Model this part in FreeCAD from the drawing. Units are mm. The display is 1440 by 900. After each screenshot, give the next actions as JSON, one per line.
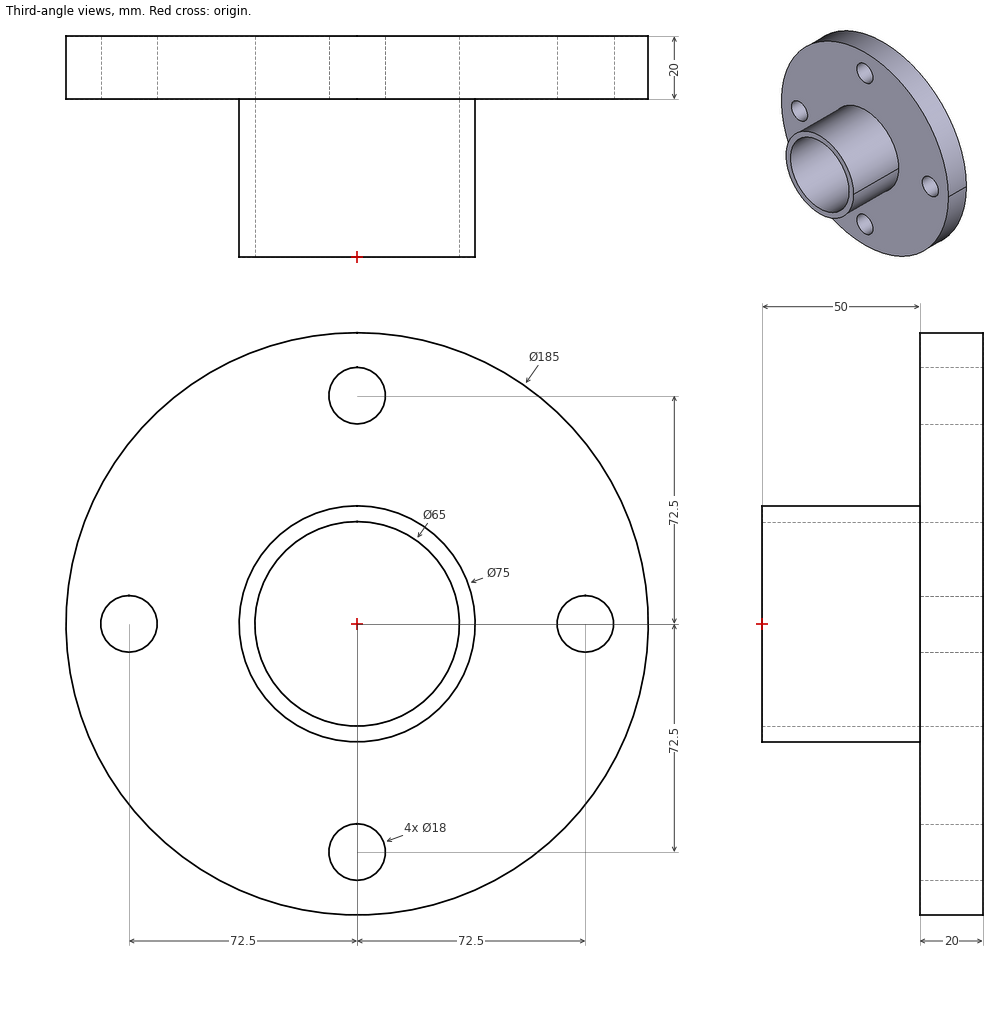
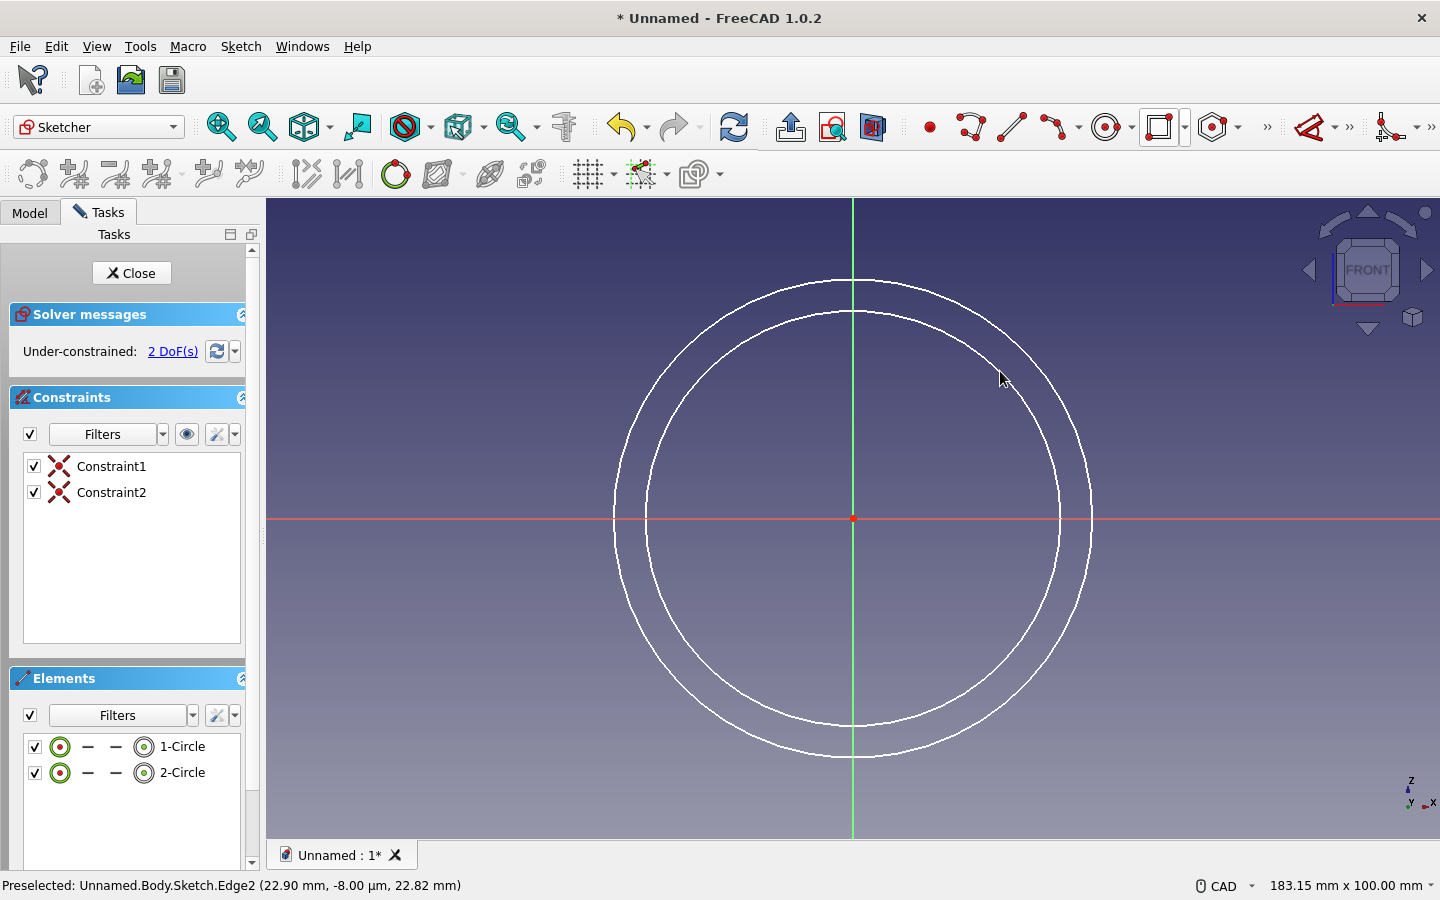
{"action": "key", "text": "d"}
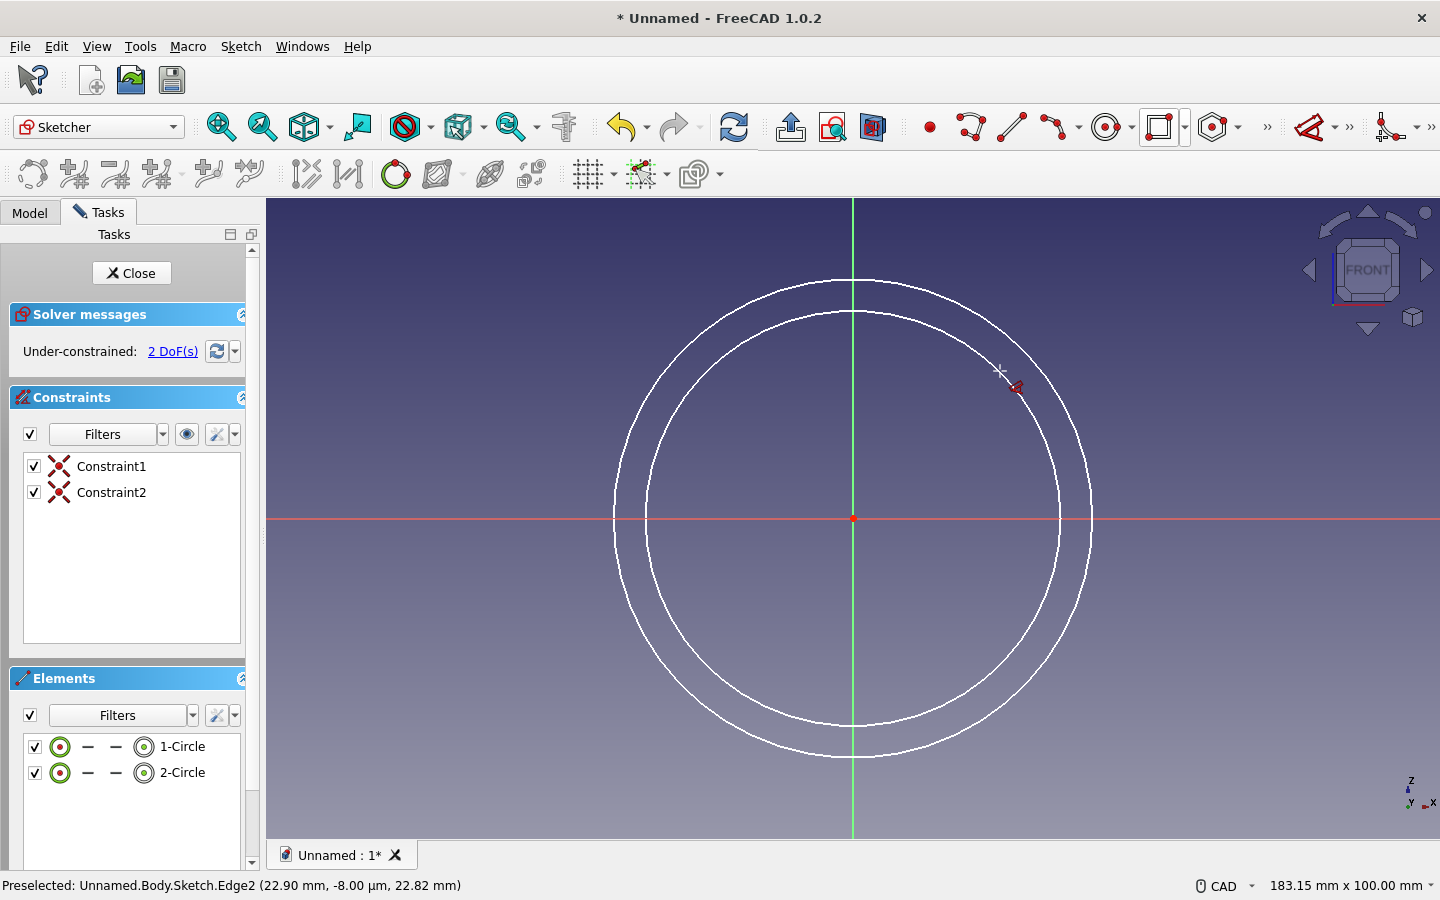
{"action": "left_click", "coordinate": [1022, 349]}
{"action": "left_click", "coordinate": [1045, 326]}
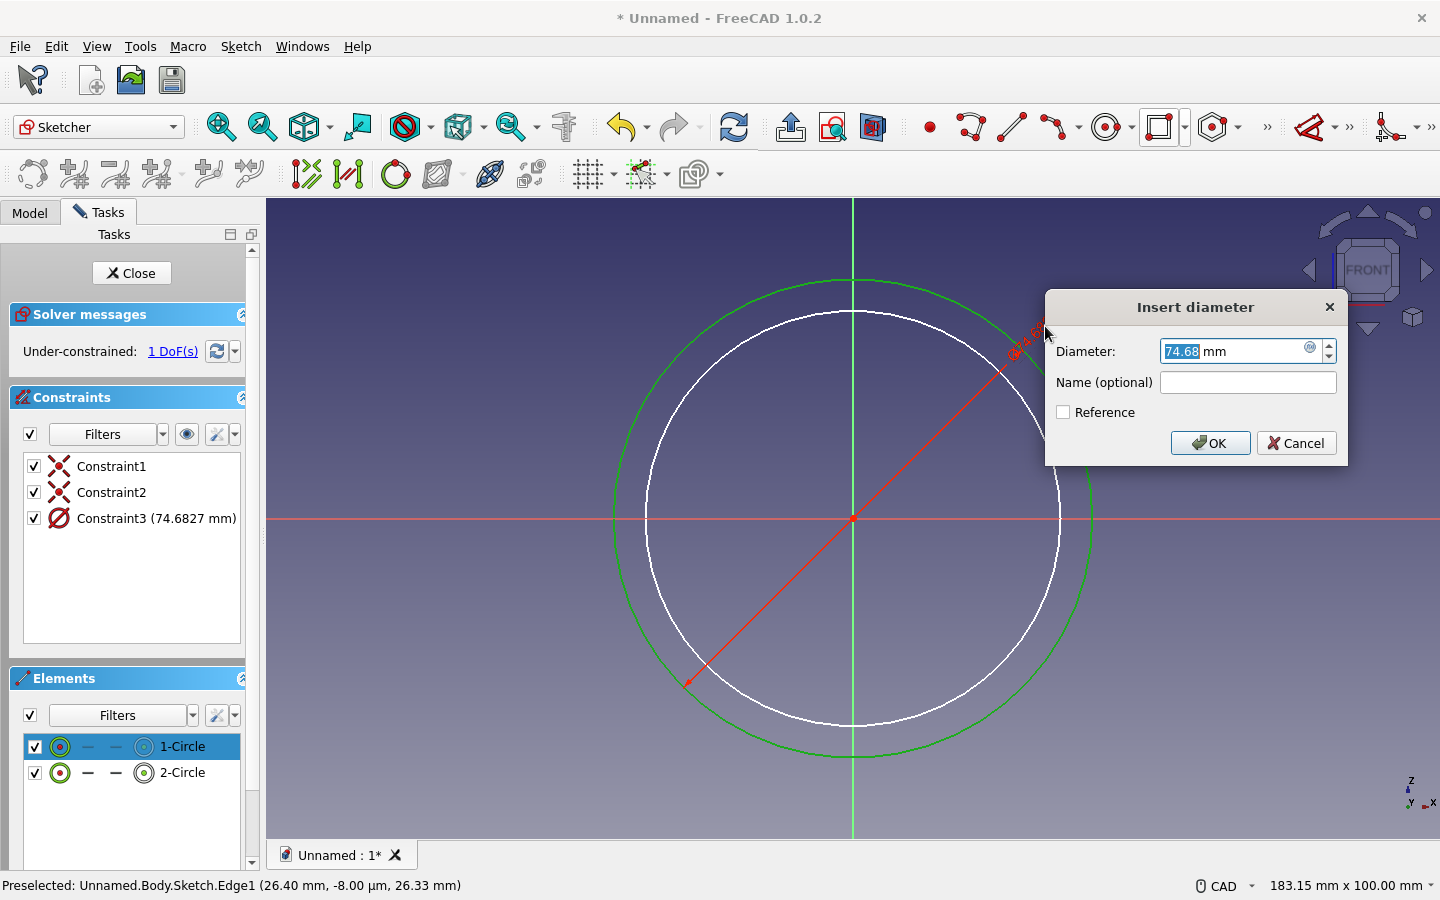
{"action": "type", "text": "75"}
{"action": "key", "text": "Return"}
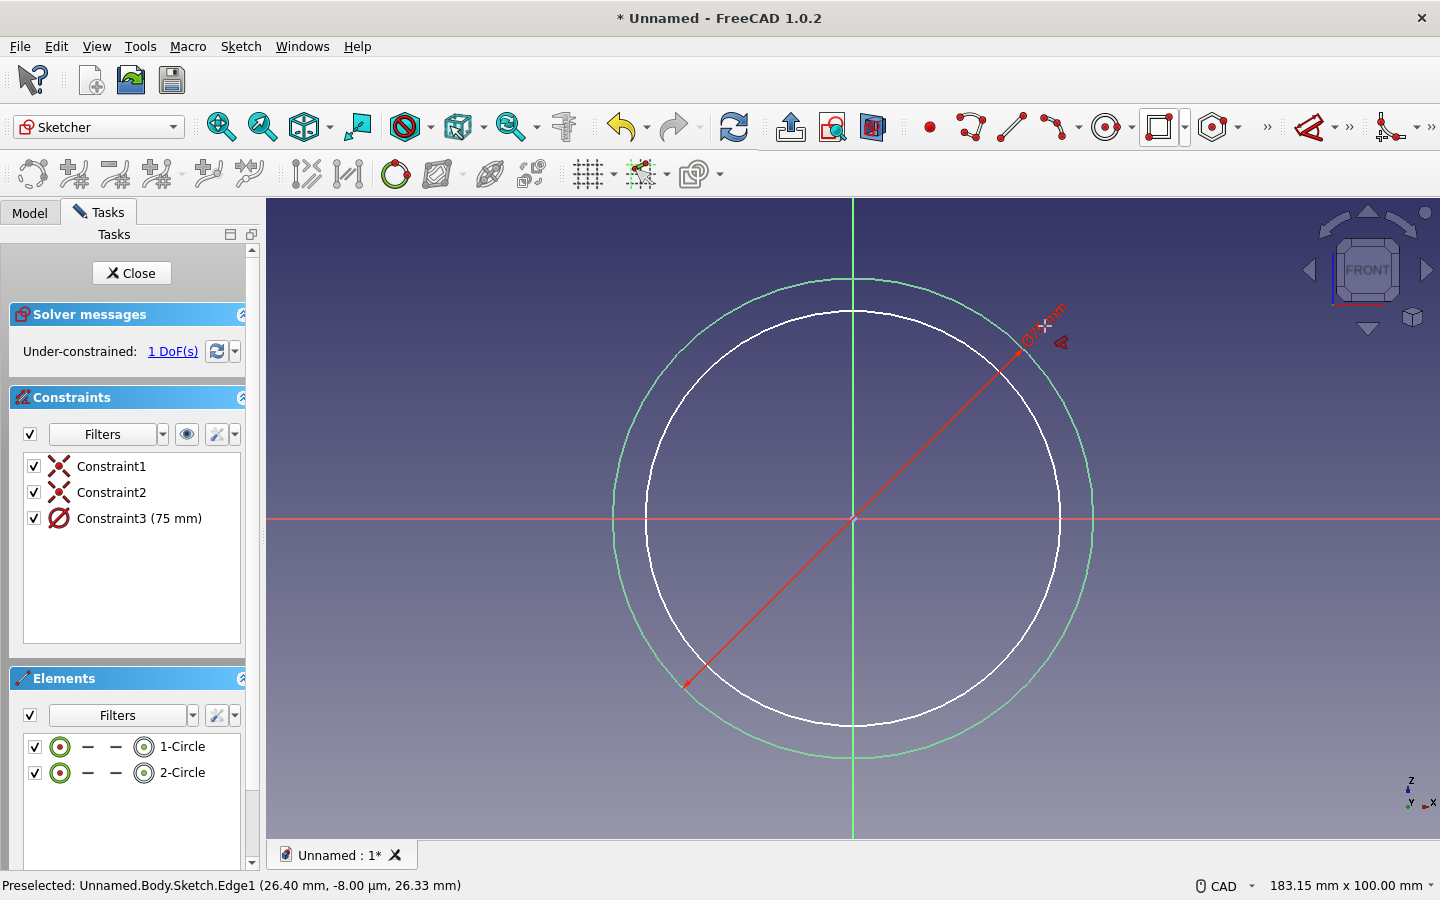
{"action": "left_click", "coordinate": [999, 371]}
{"action": "left_click", "coordinate": [1105, 443]}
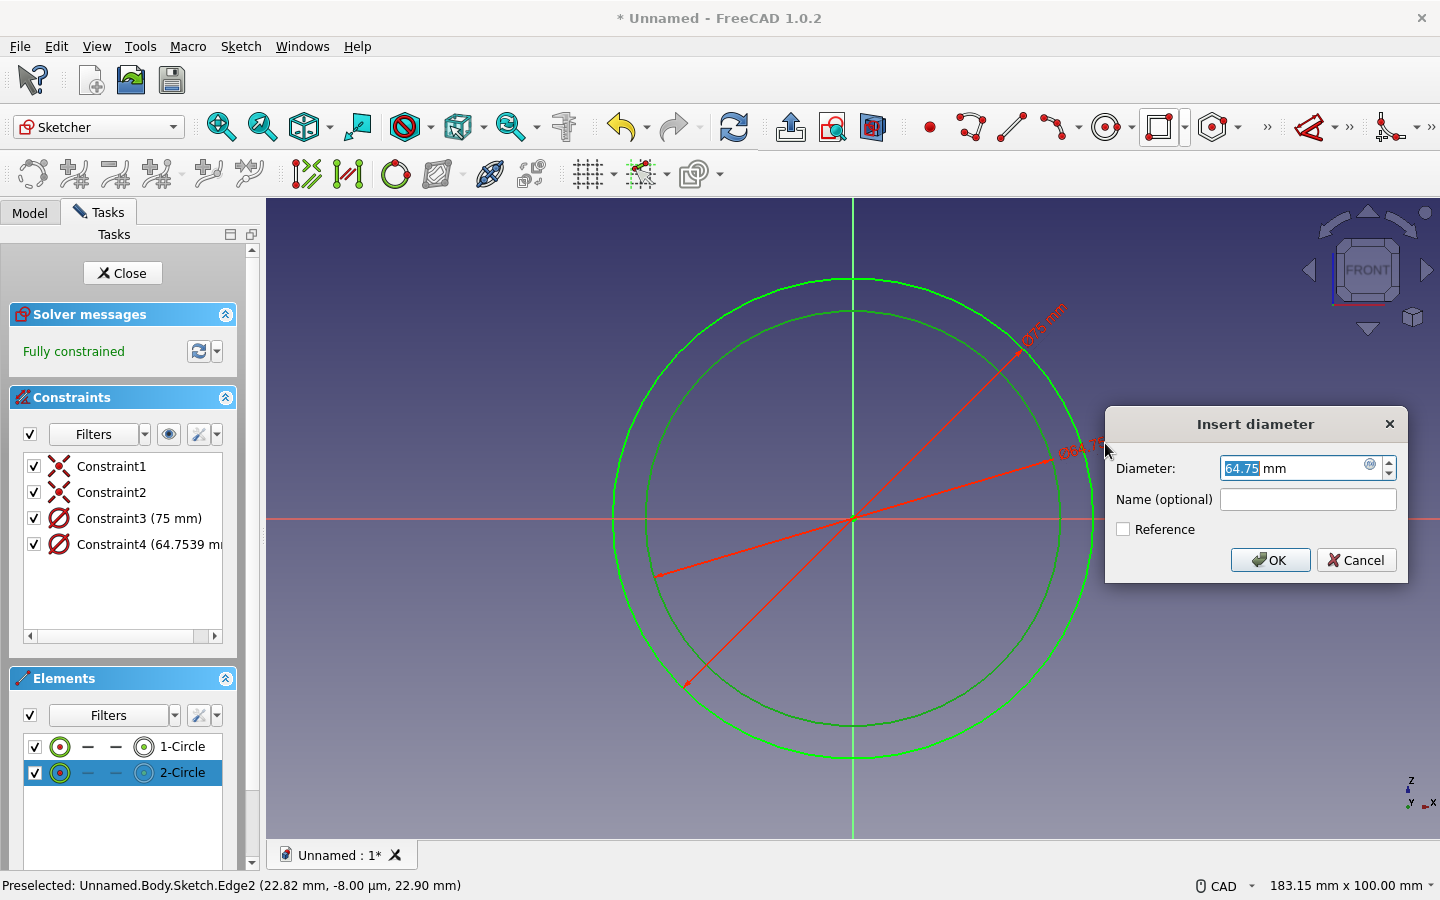
{"action": "type", "text": "65"}
{"action": "key", "text": "Return"}
{"action": "key", "text": "Escape"}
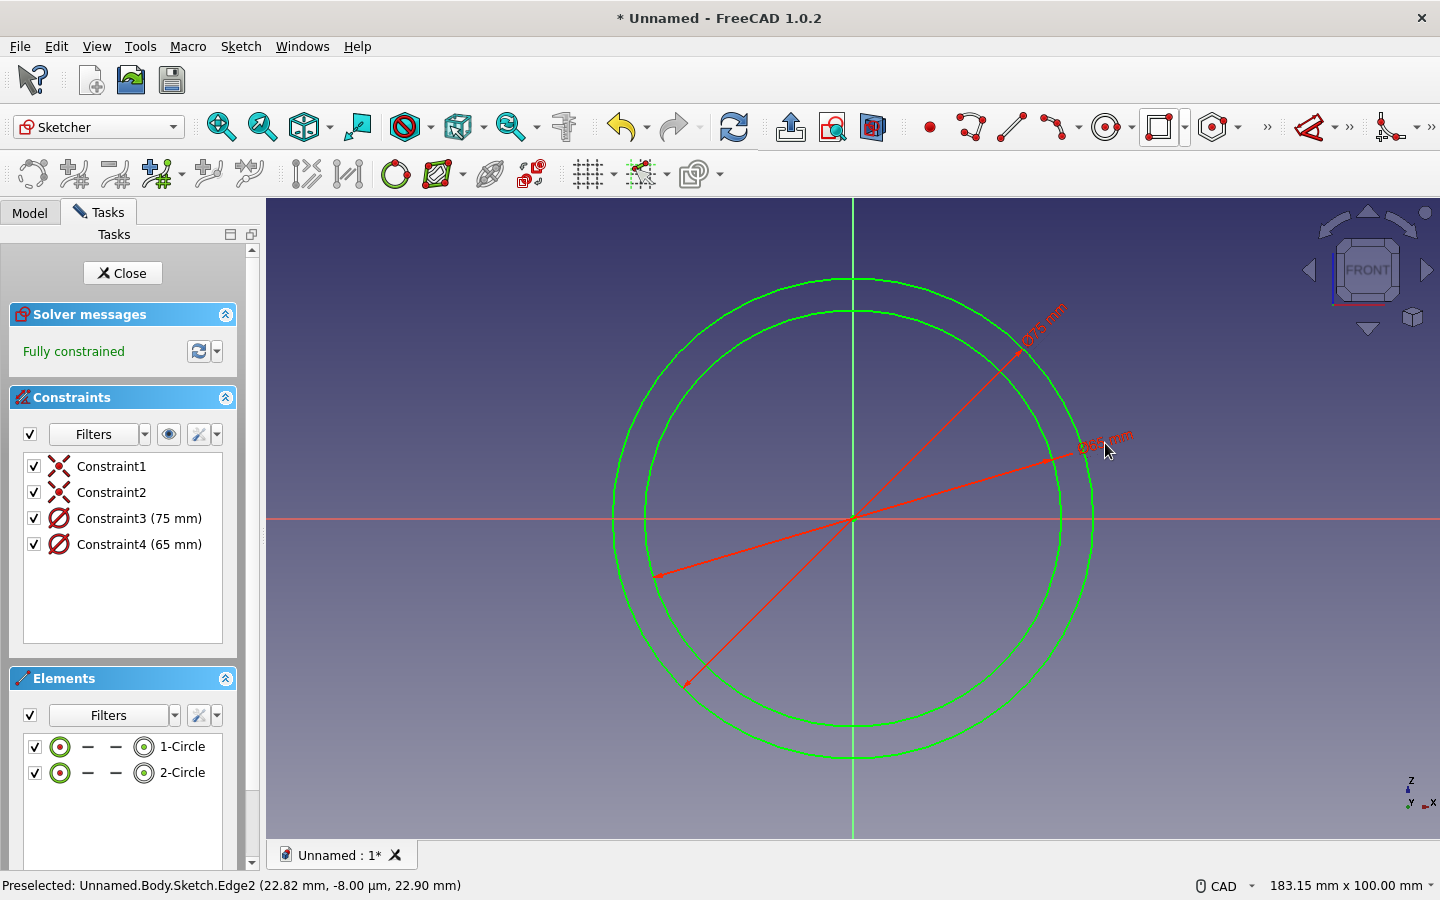
{"action": "left_click", "coordinate": [123, 273]}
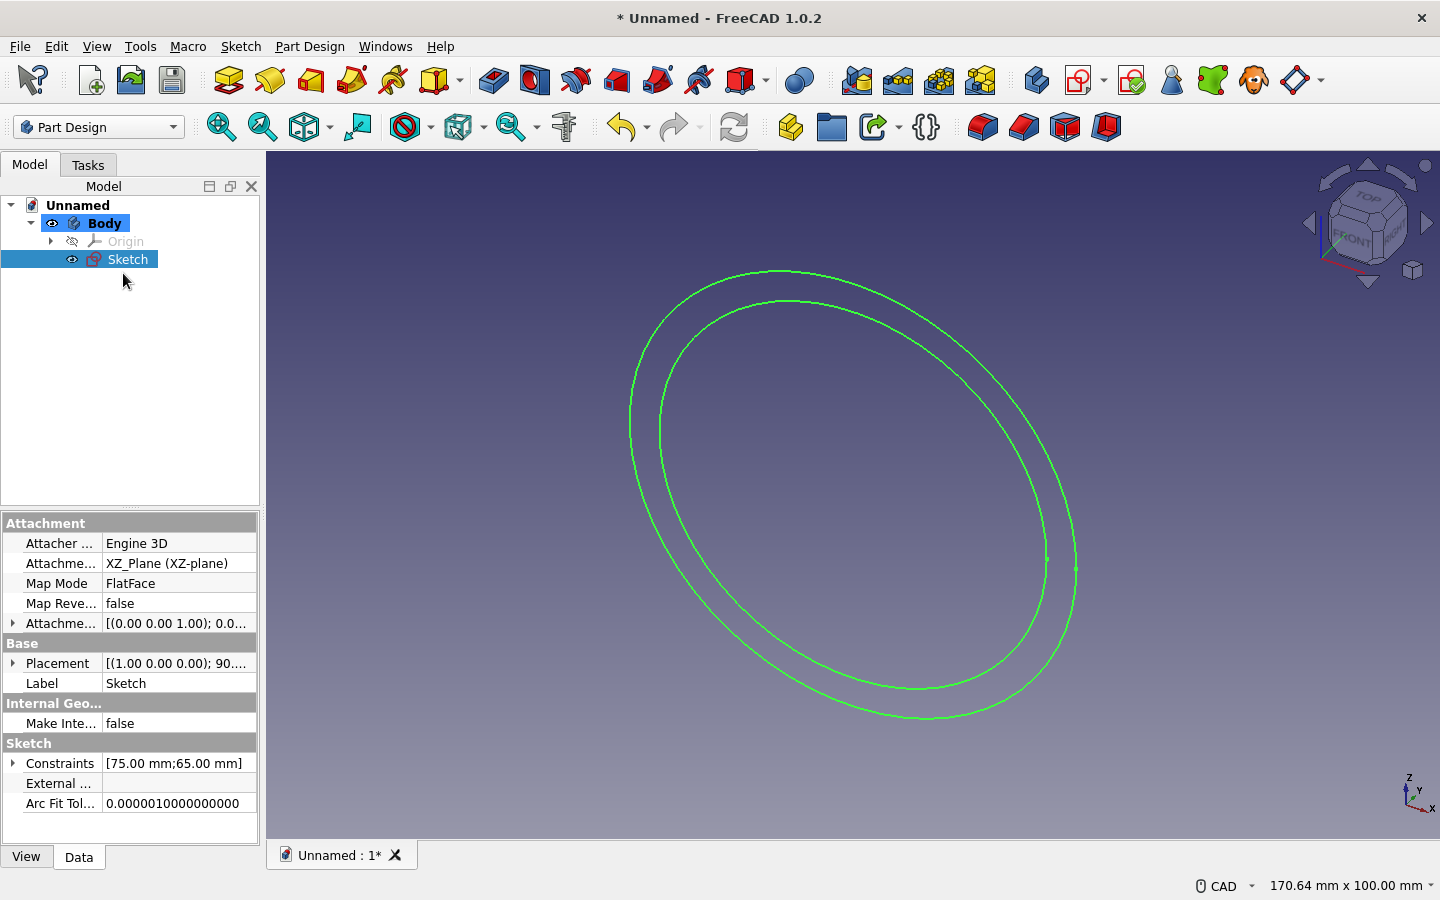
{"action": "left_click", "coordinate": [229, 80]}